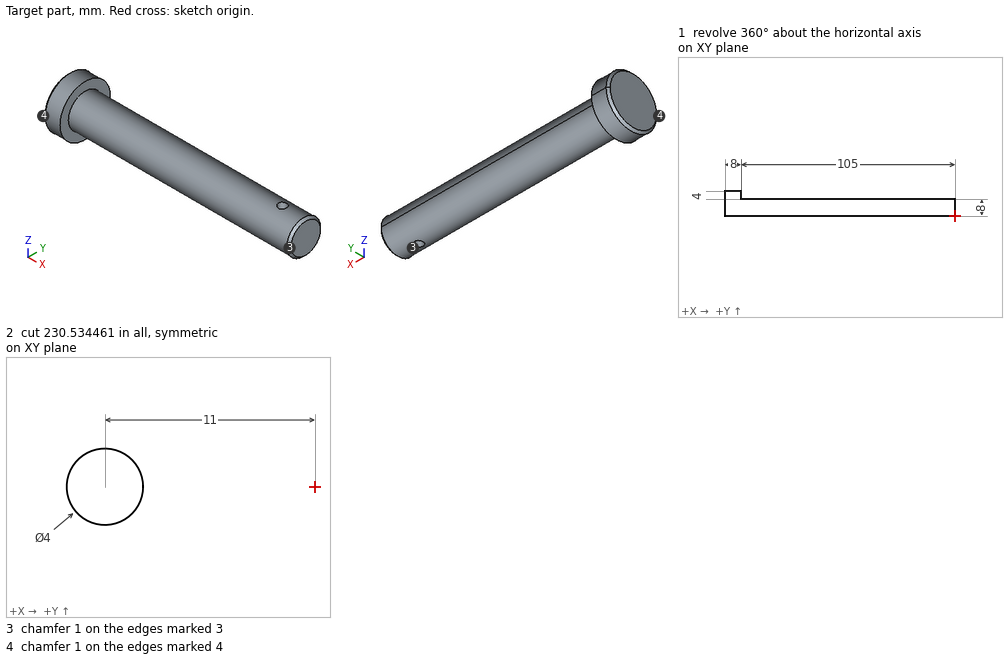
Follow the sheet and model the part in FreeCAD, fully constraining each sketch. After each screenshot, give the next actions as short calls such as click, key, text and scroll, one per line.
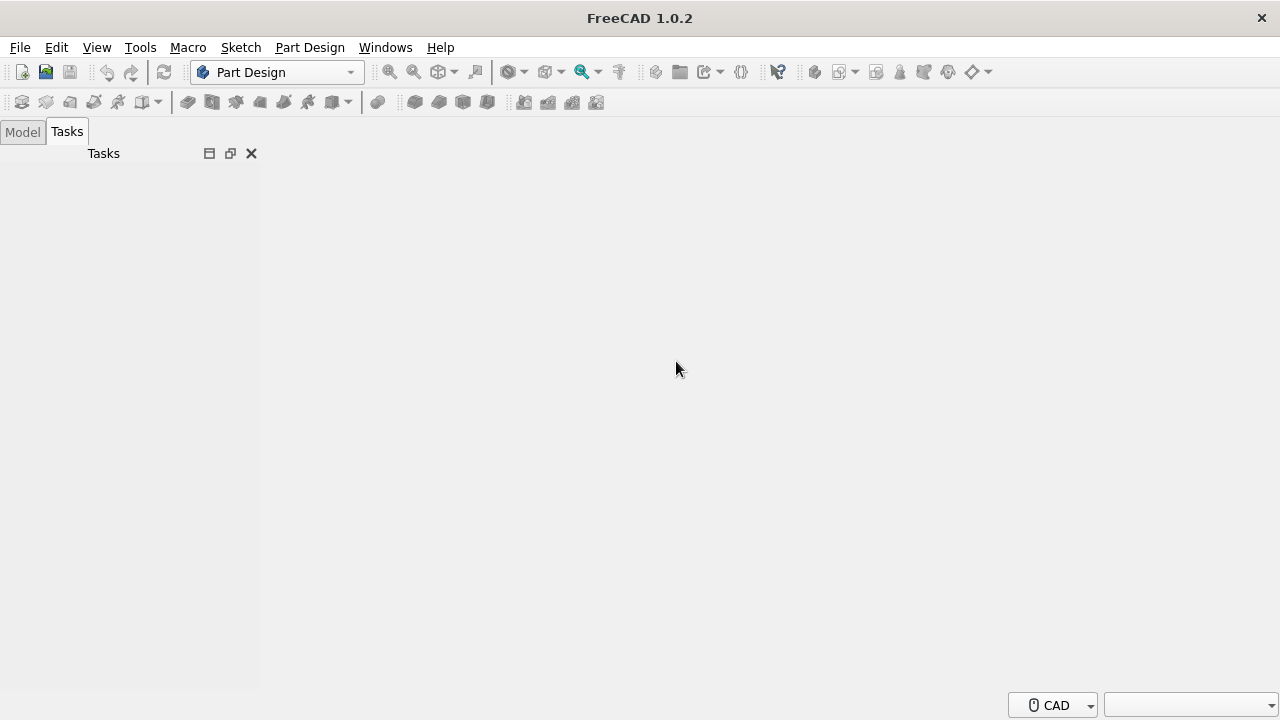
click(22, 72)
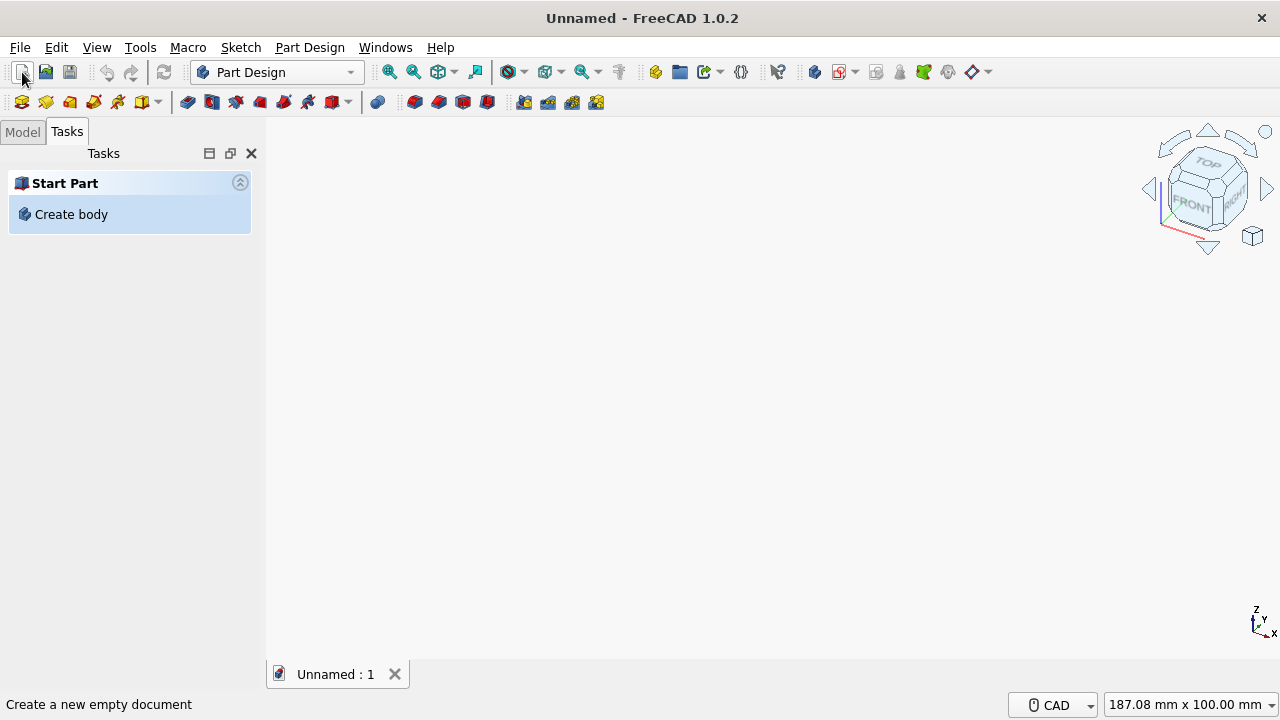
click(840, 72)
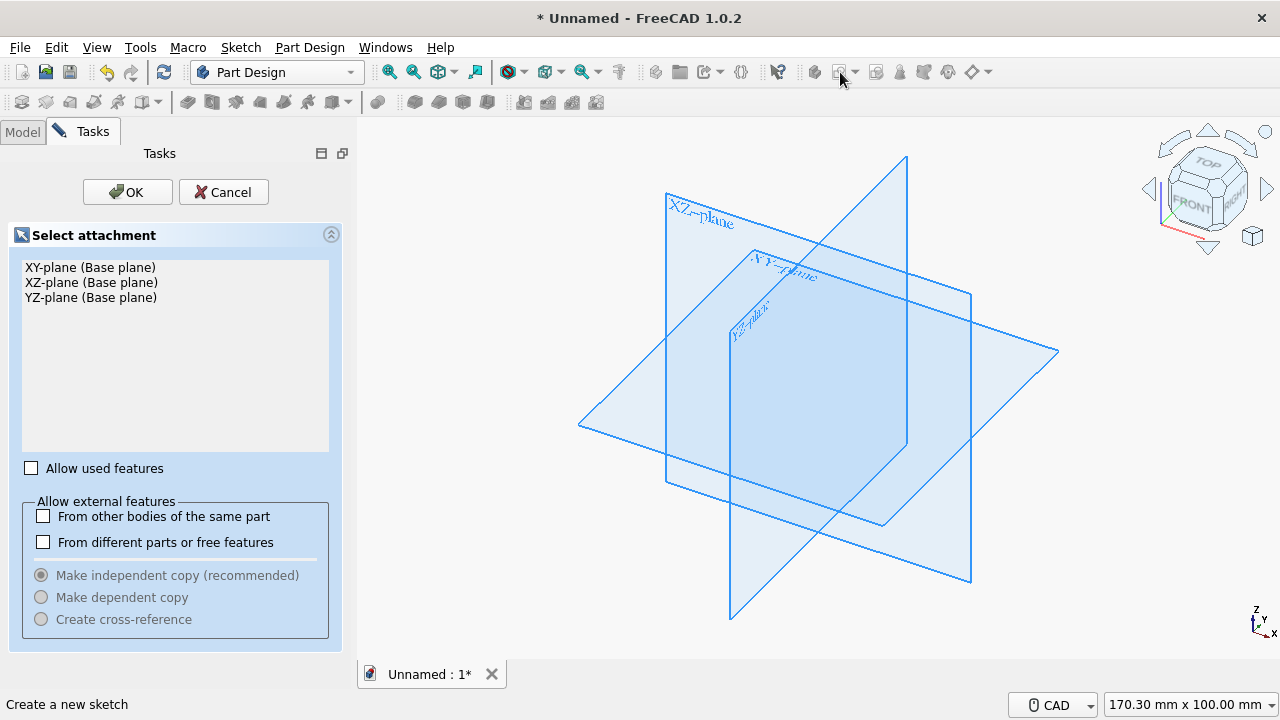
click(82, 268)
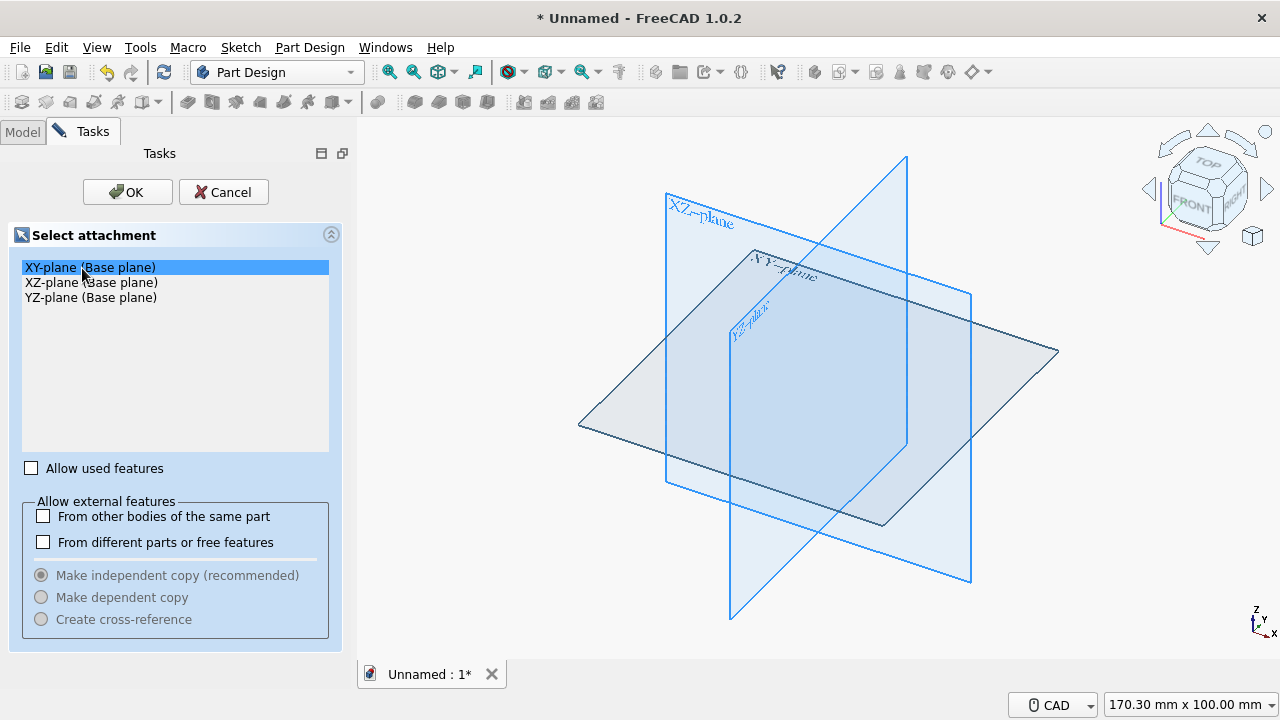
click(128, 192)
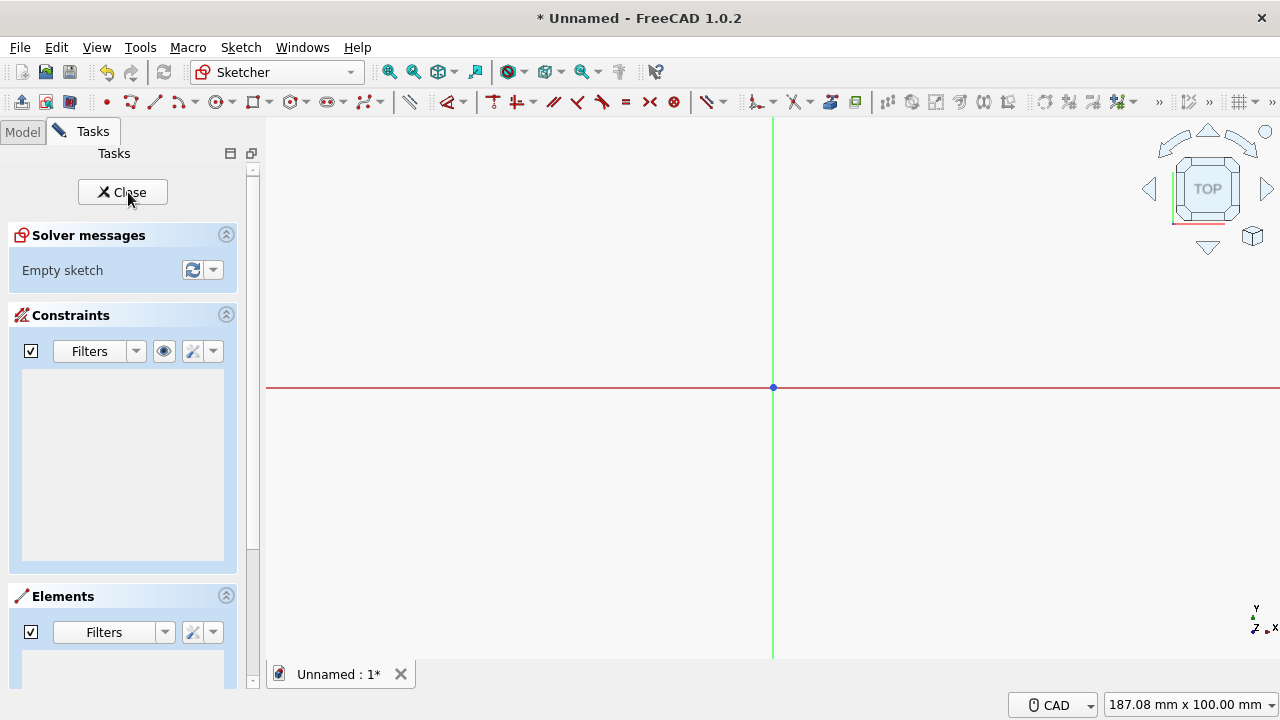
scroll(1115, 535, down, 1)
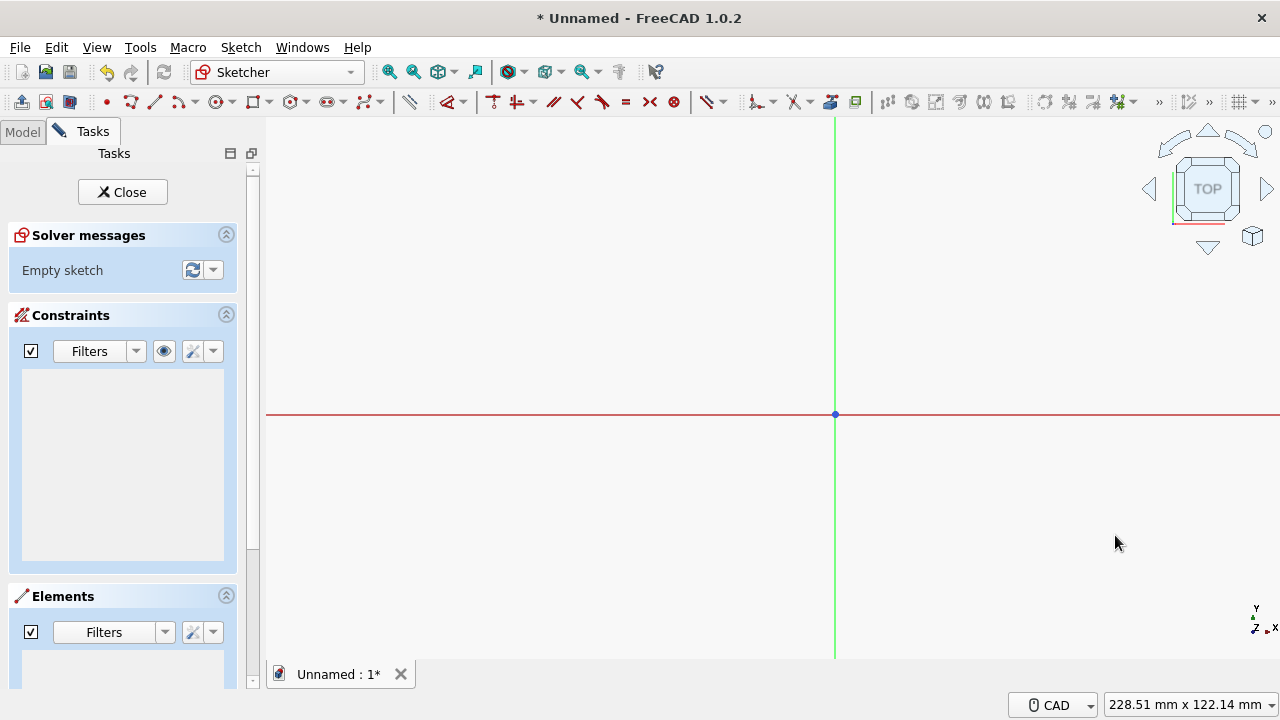
click(132, 102)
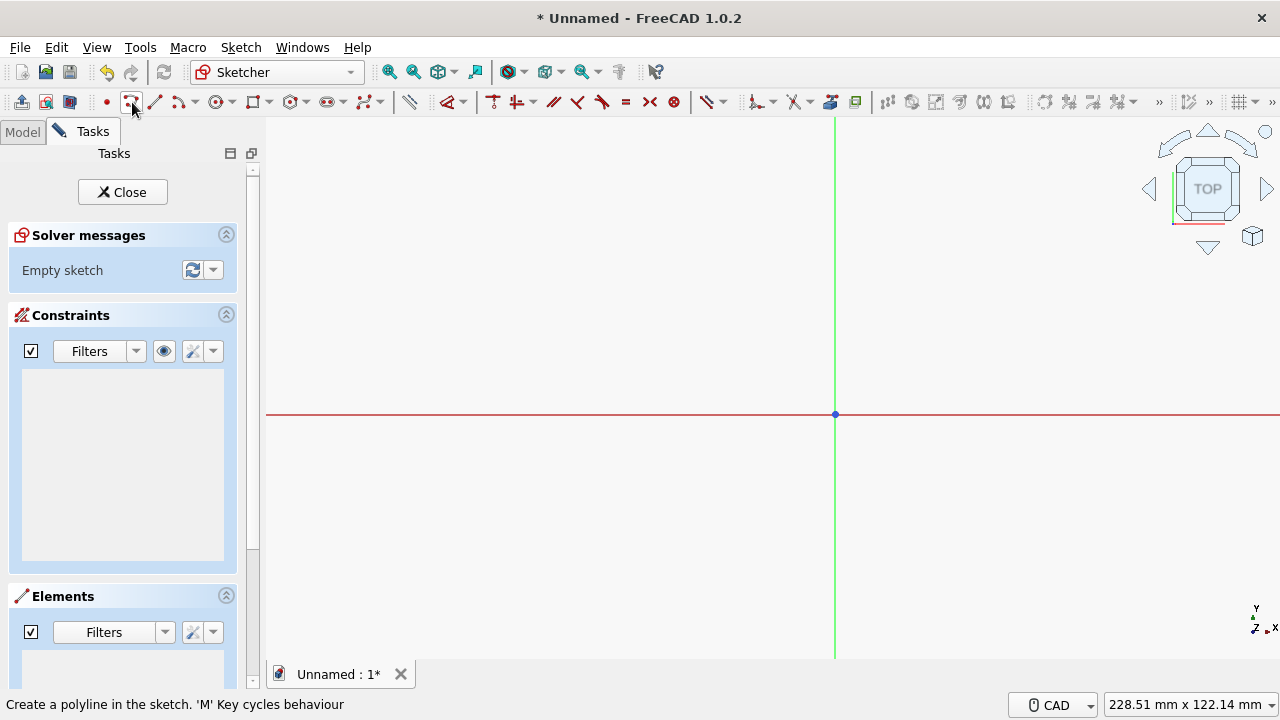
click(835, 415)
click(826, 379)
click(369, 379)
click(369, 362)
click(334, 362)
click(334, 406)
click(835, 415)
key(Escape)
key(Escape)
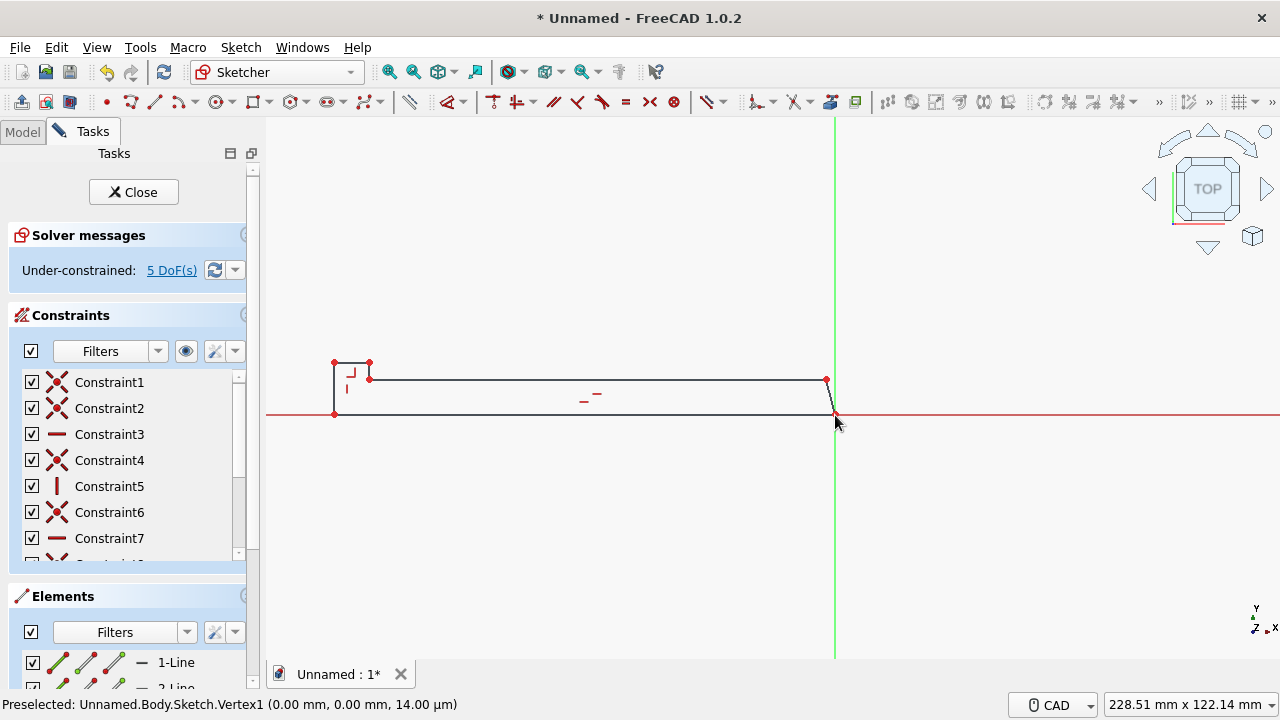
scroll(832, 404, up, 2)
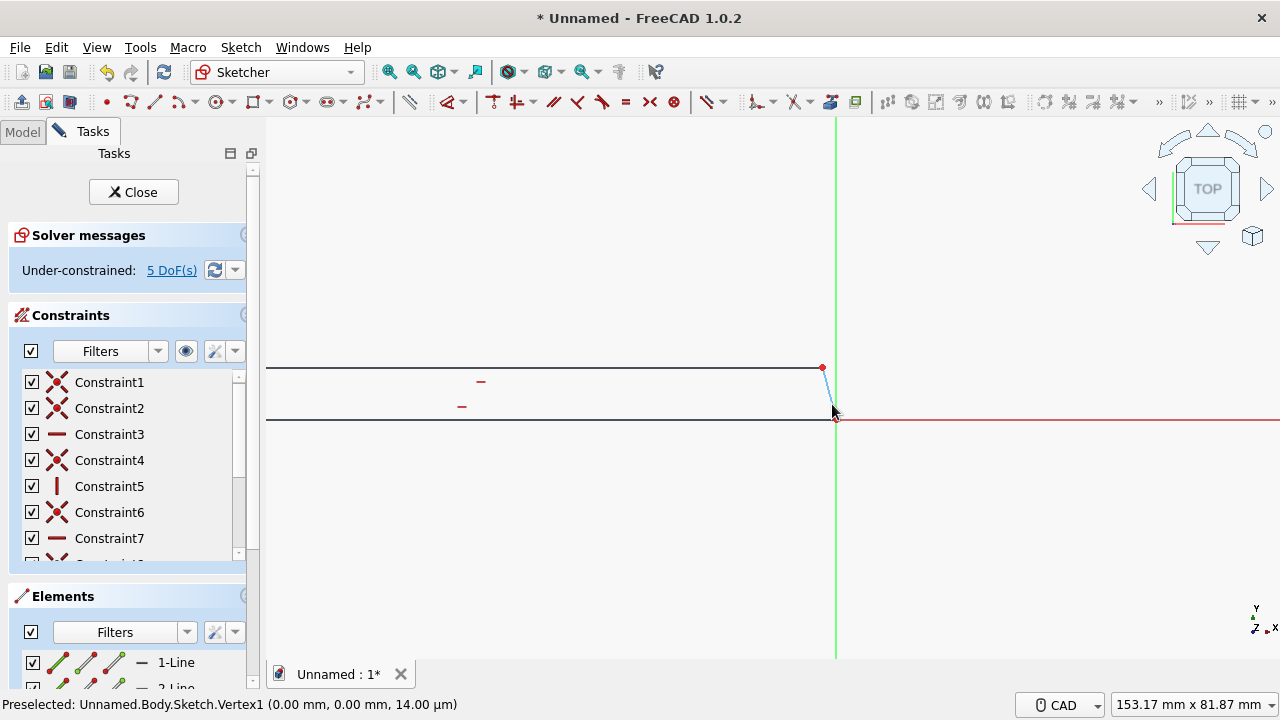
click(832, 404)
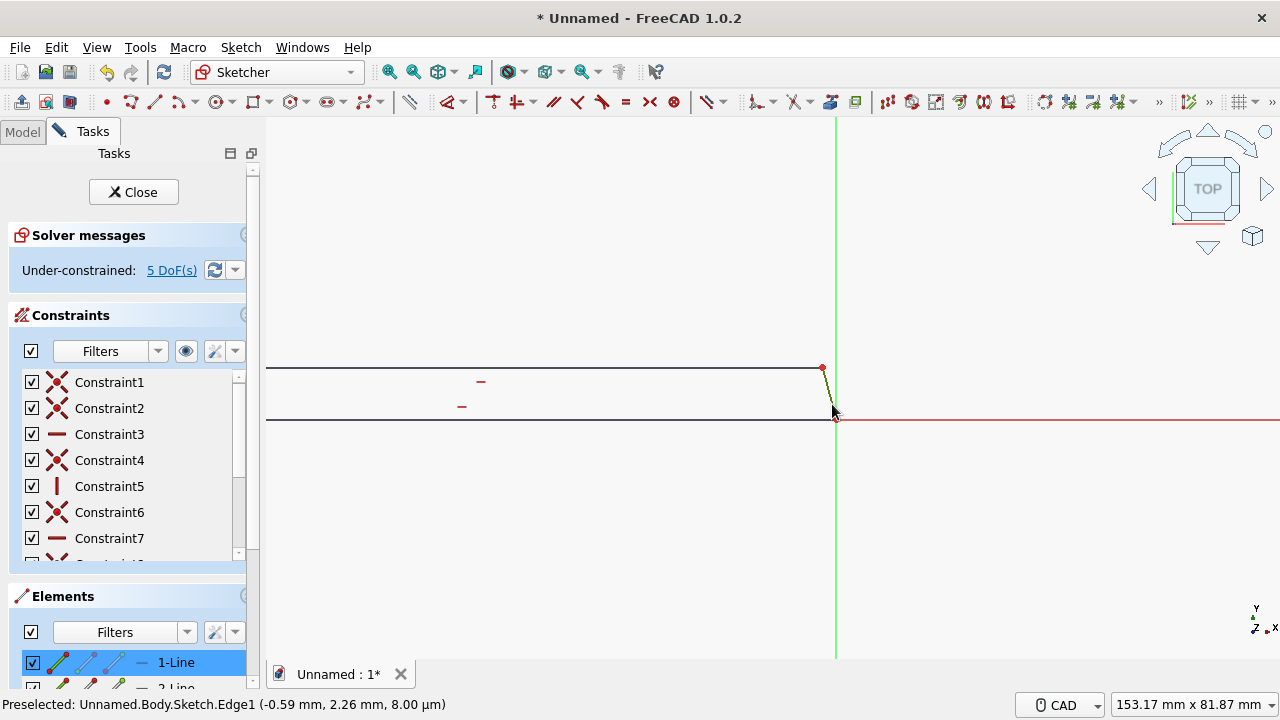
click(536, 102)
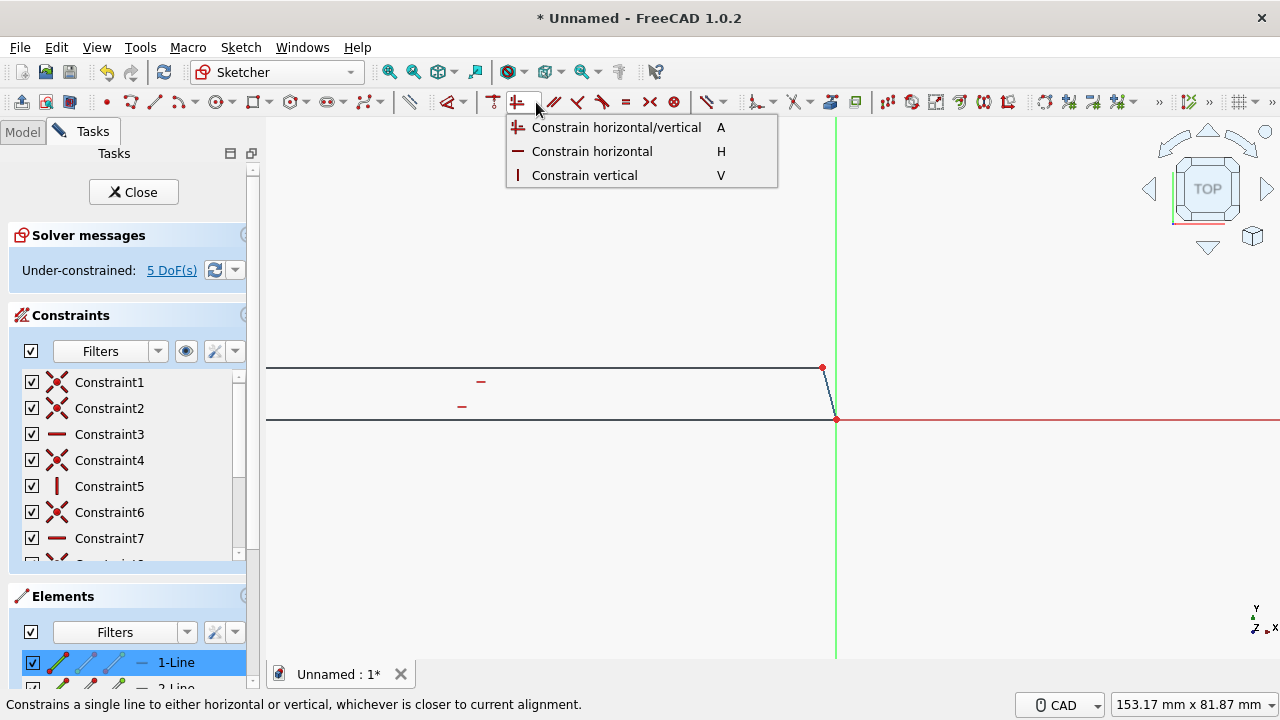
click(642, 175)